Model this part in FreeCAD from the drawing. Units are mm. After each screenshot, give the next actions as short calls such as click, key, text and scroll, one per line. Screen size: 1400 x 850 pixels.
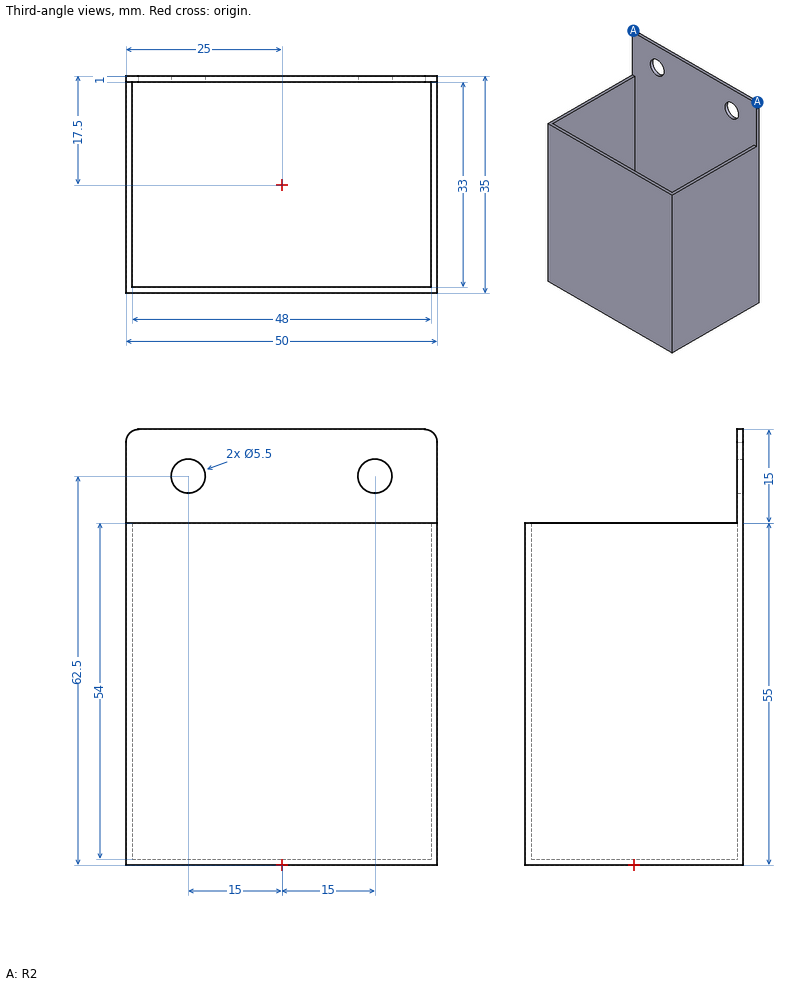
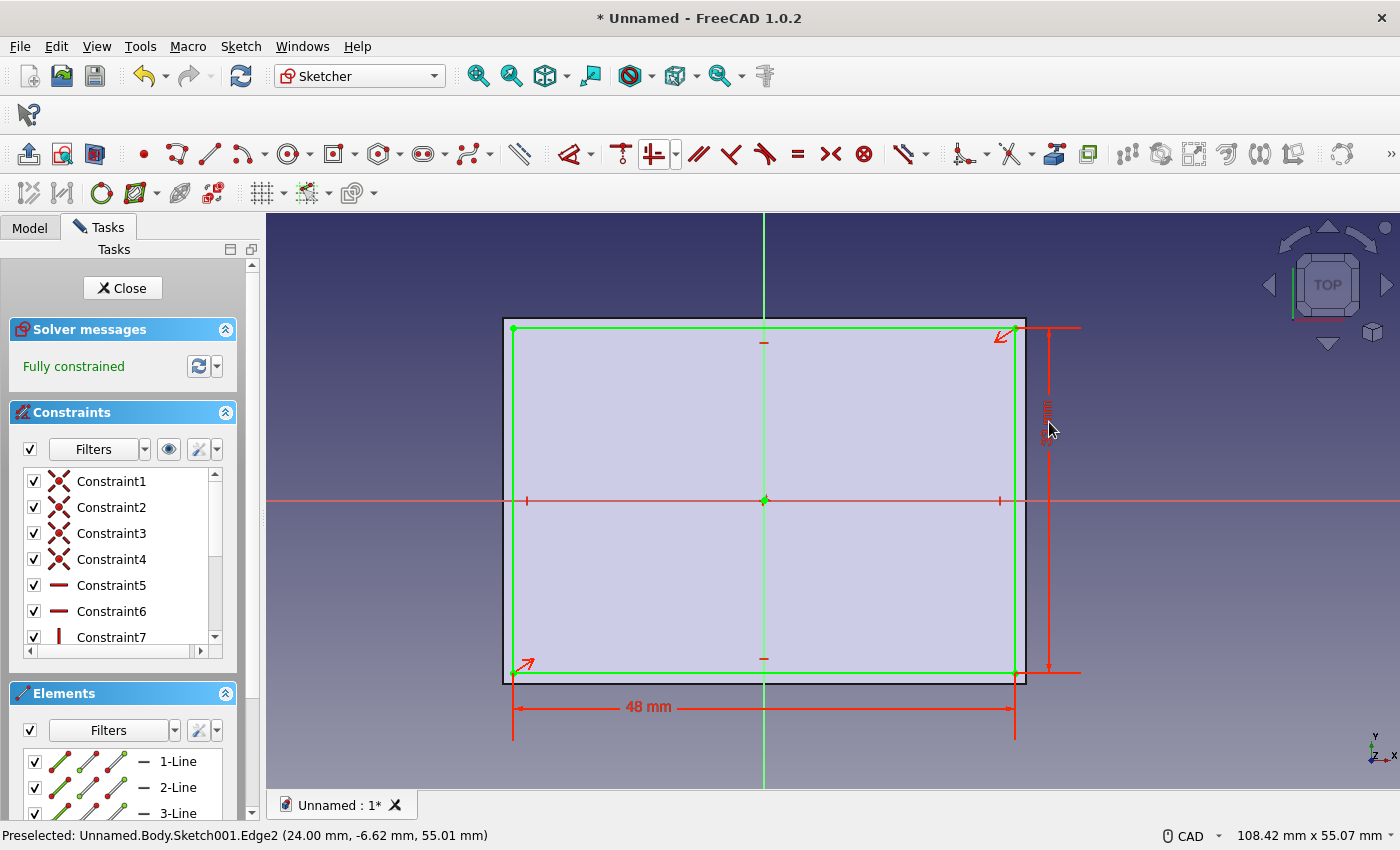
click(123, 288)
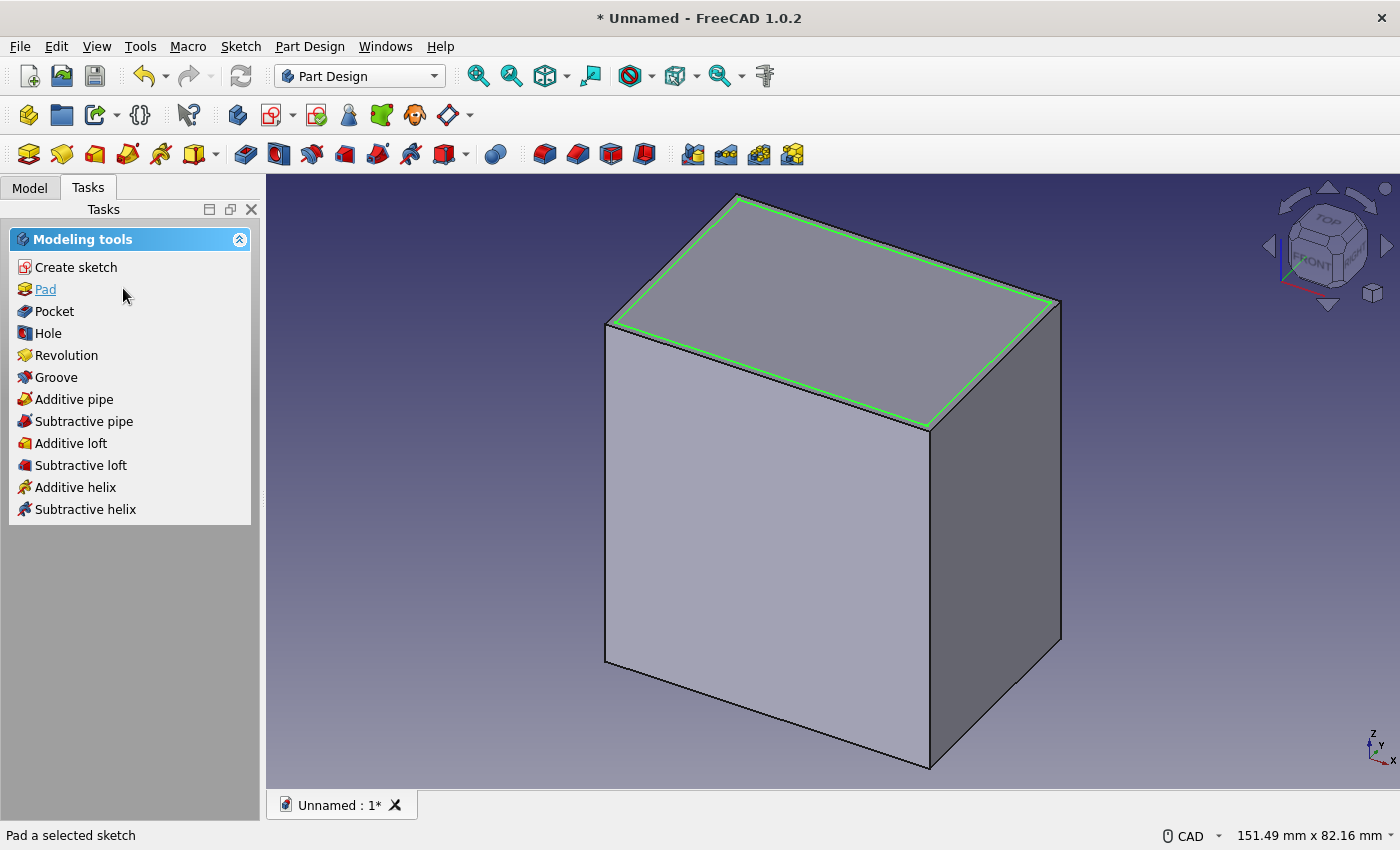
click(246, 154)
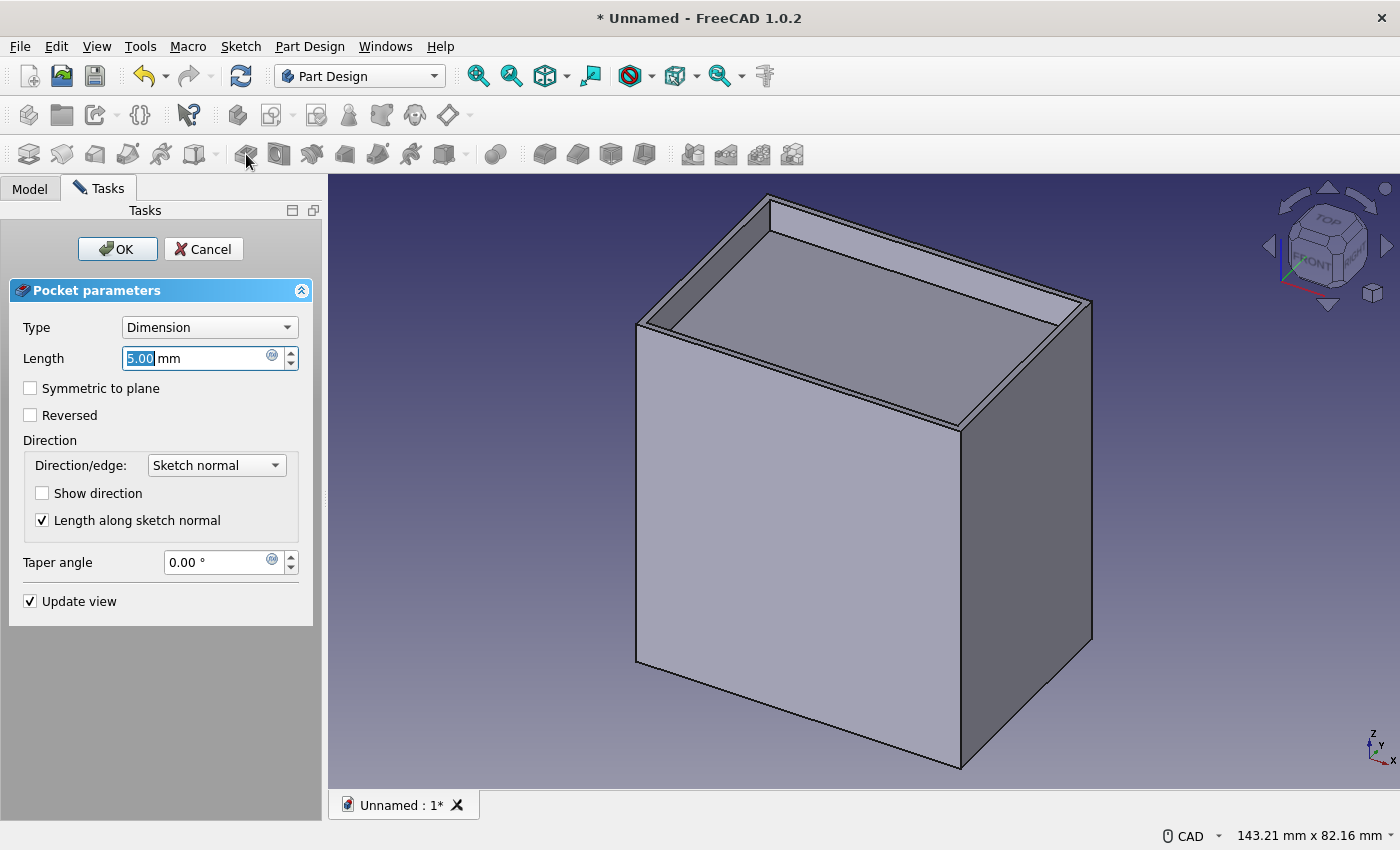
text(54)
key(Tab)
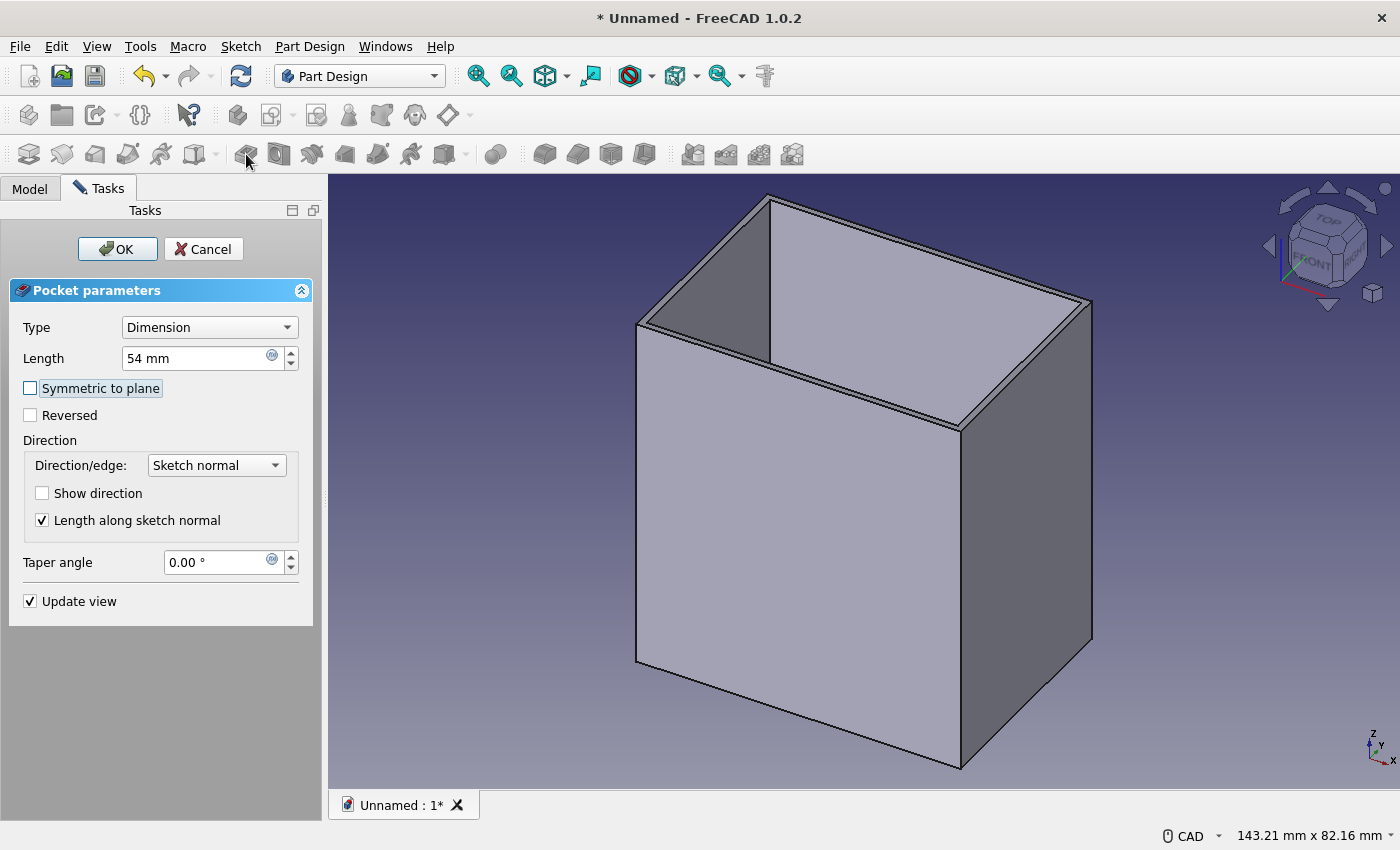
click(118, 249)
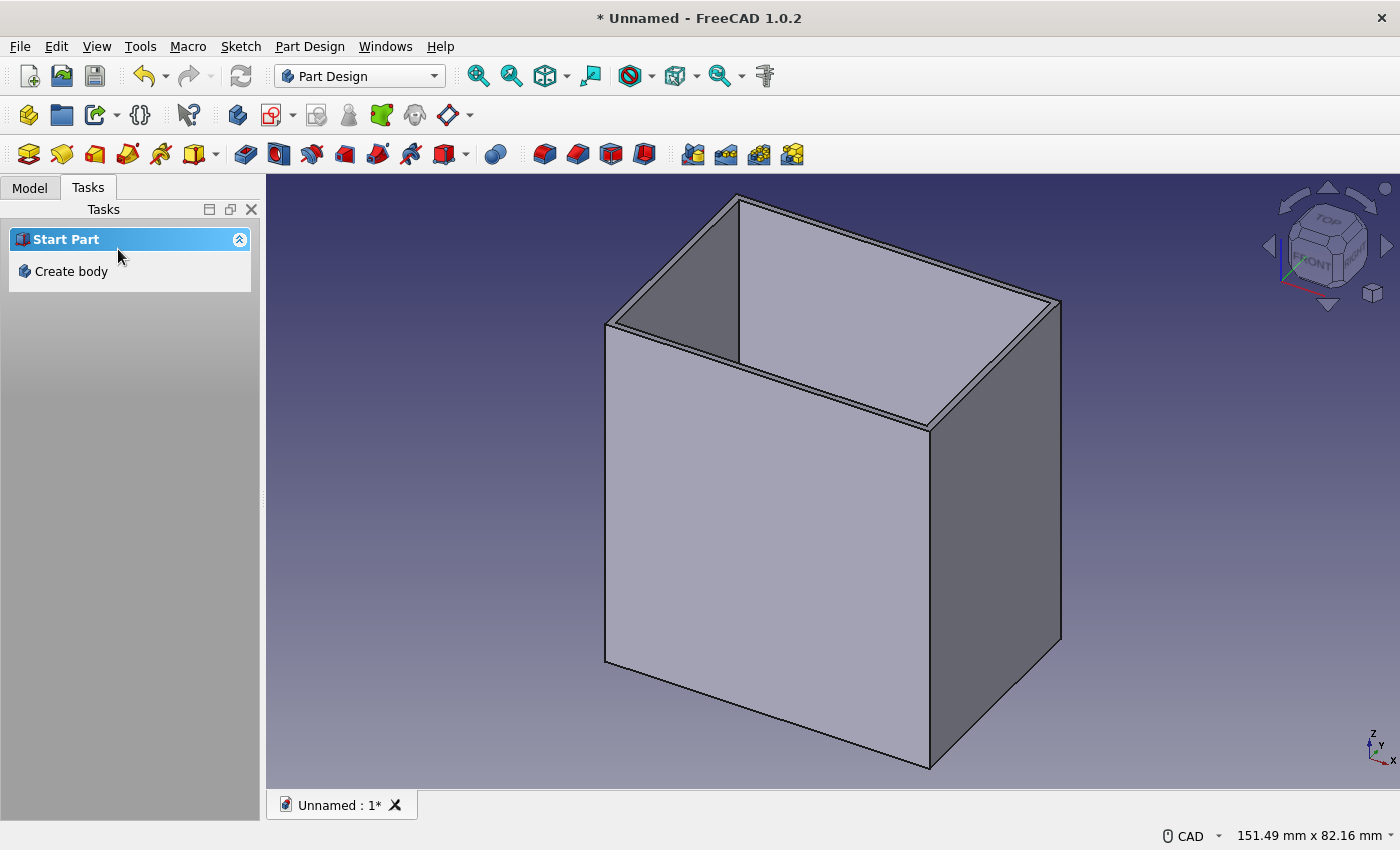
scroll(972, 385, up, 8)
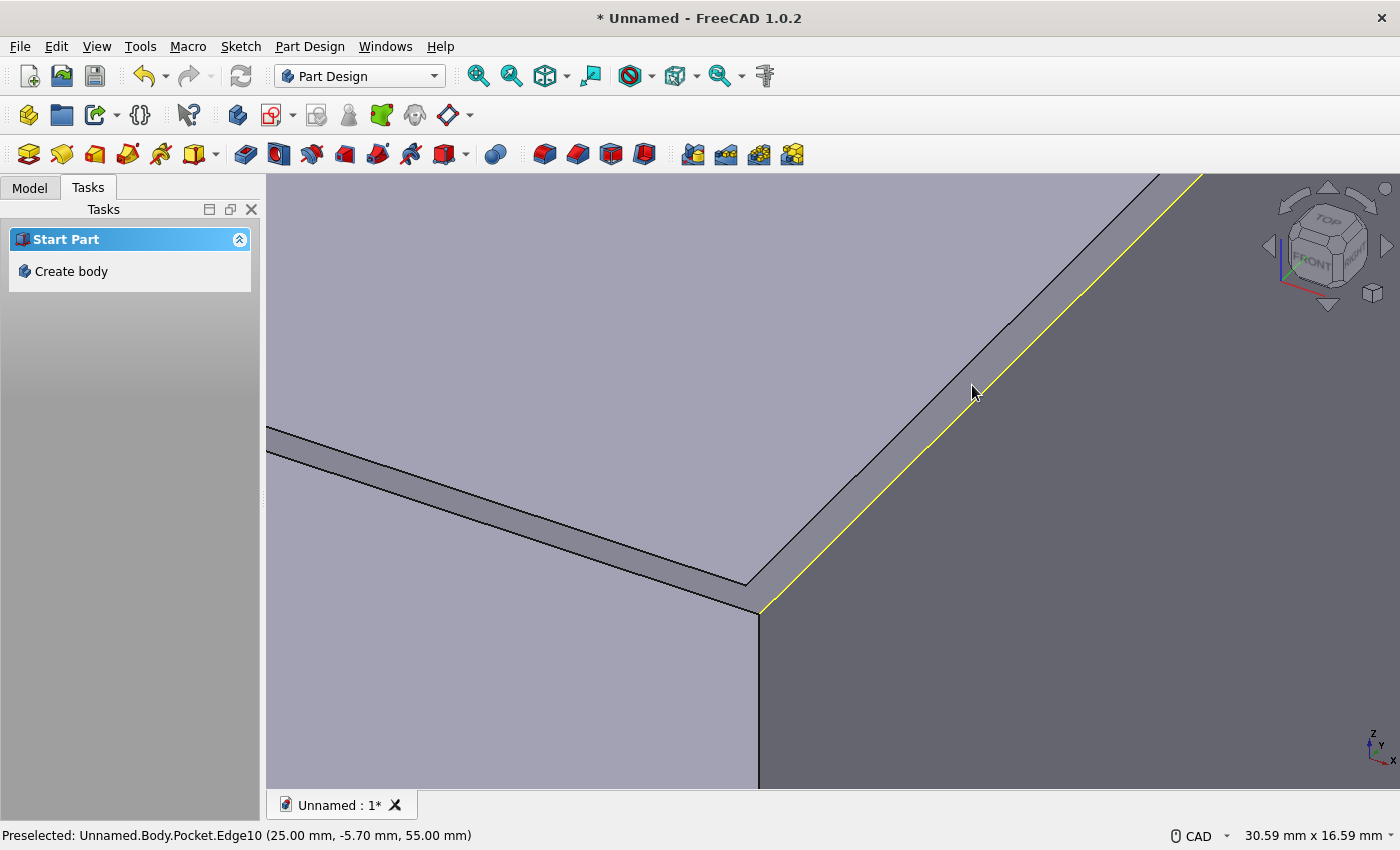
click(971, 389)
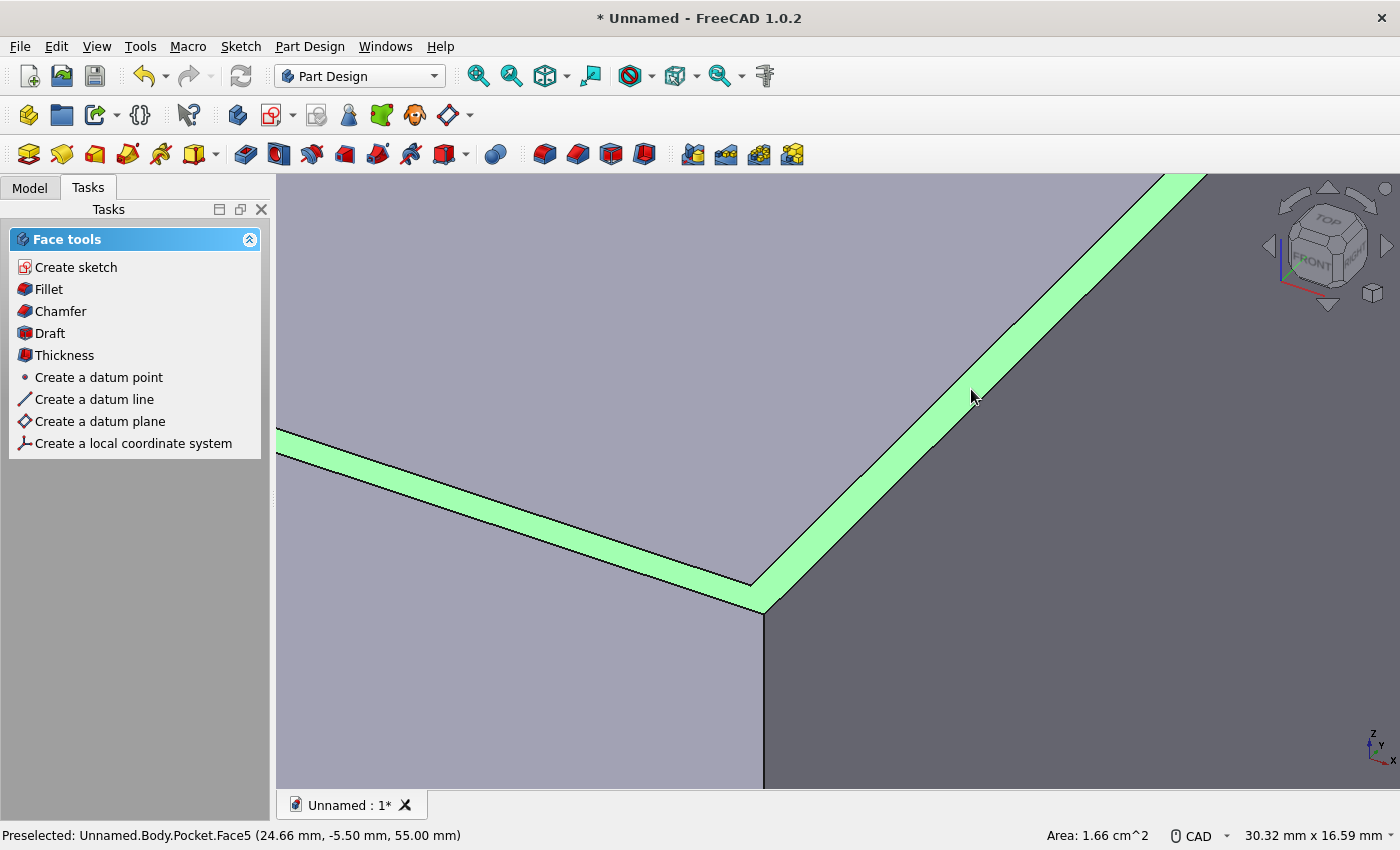
click(270, 116)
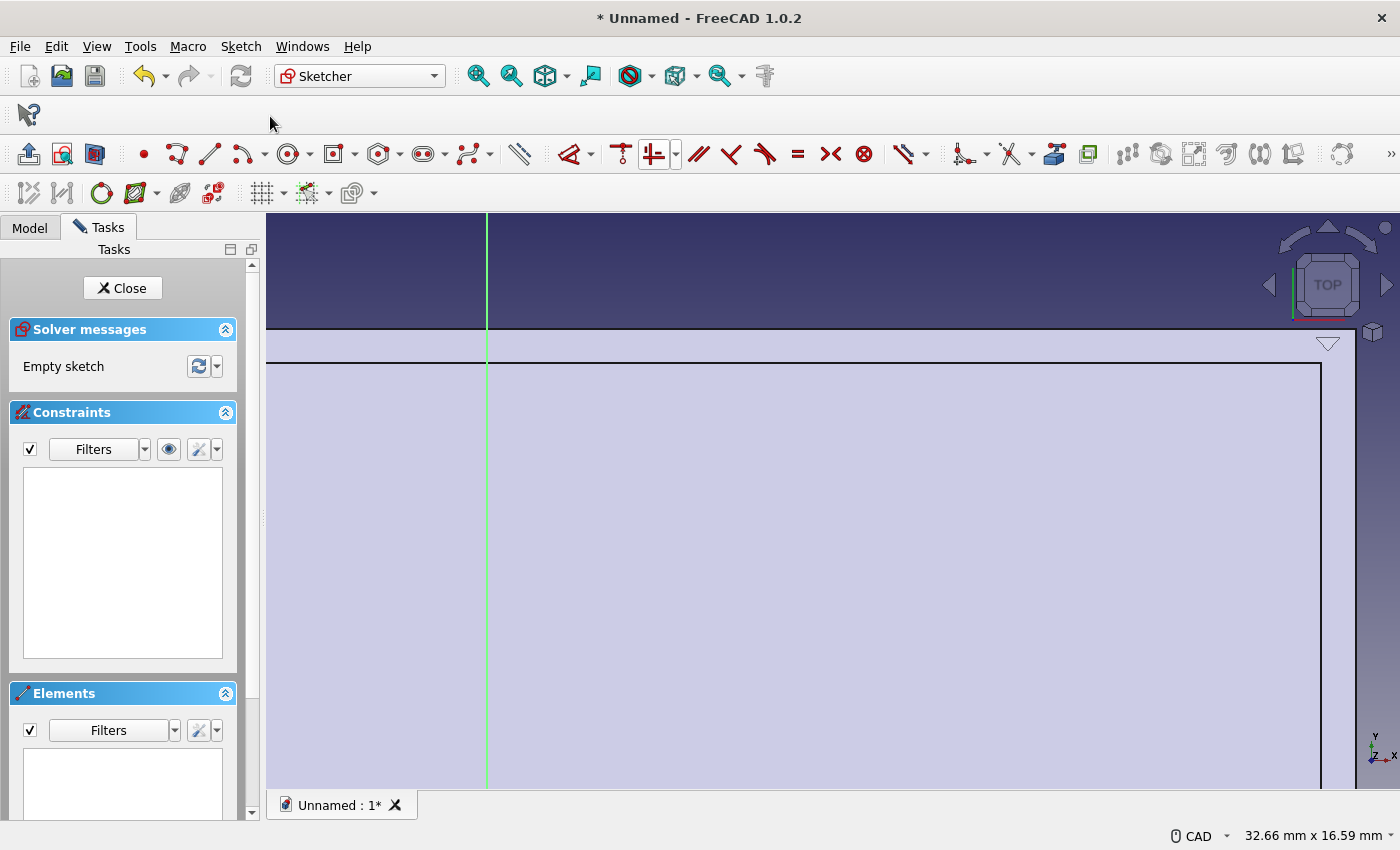
scroll(926, 424, down, 5)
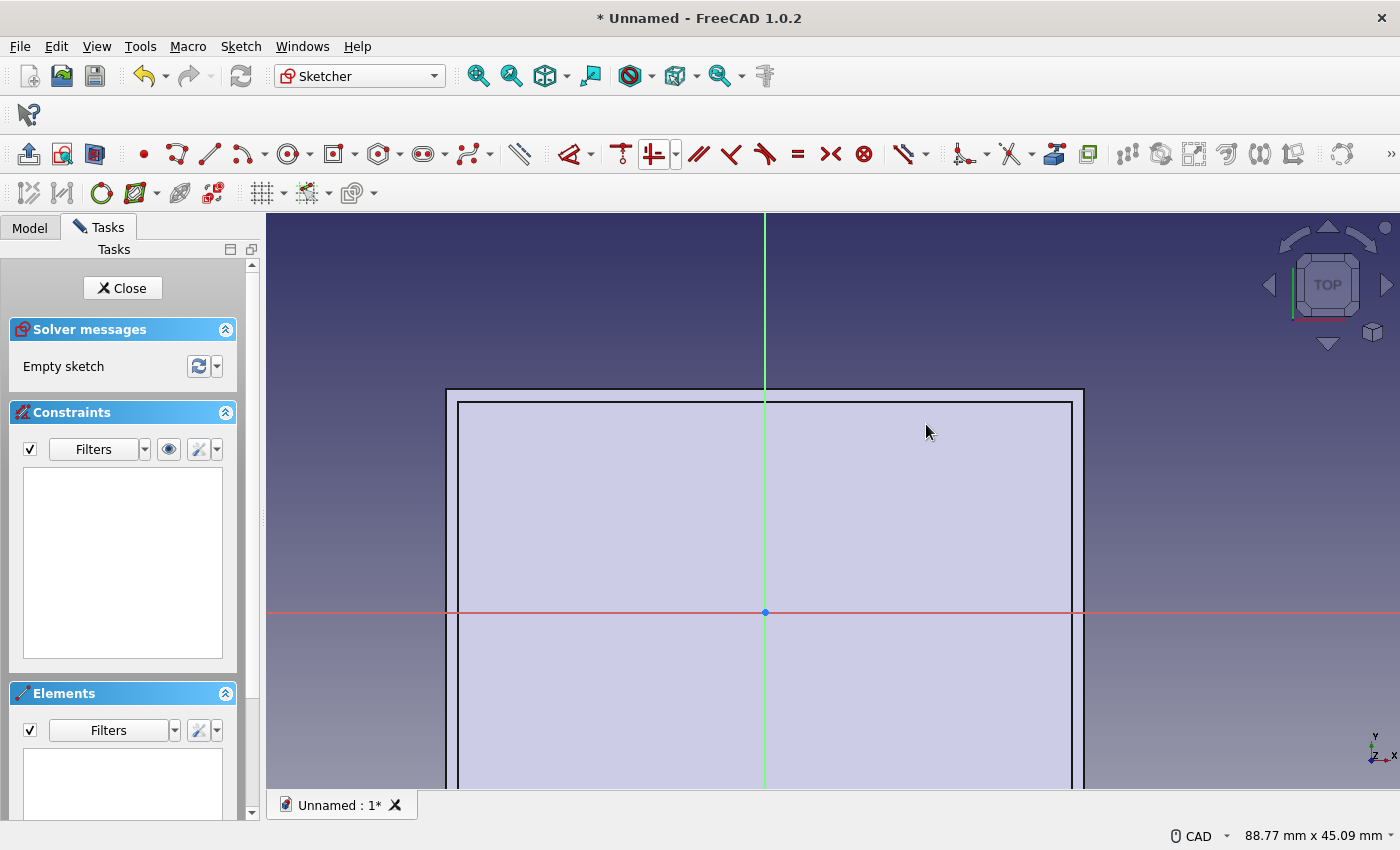
key(g)
key(r)